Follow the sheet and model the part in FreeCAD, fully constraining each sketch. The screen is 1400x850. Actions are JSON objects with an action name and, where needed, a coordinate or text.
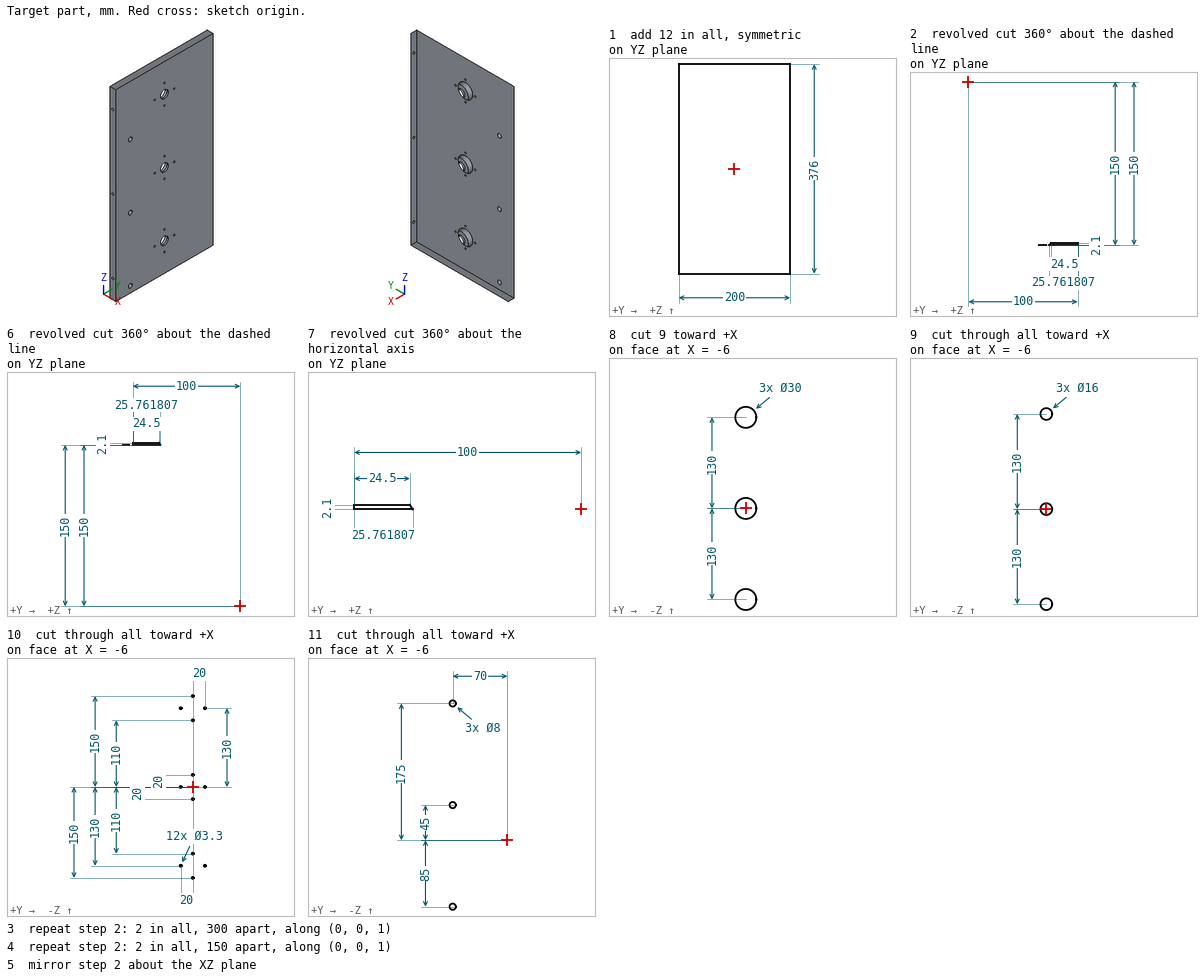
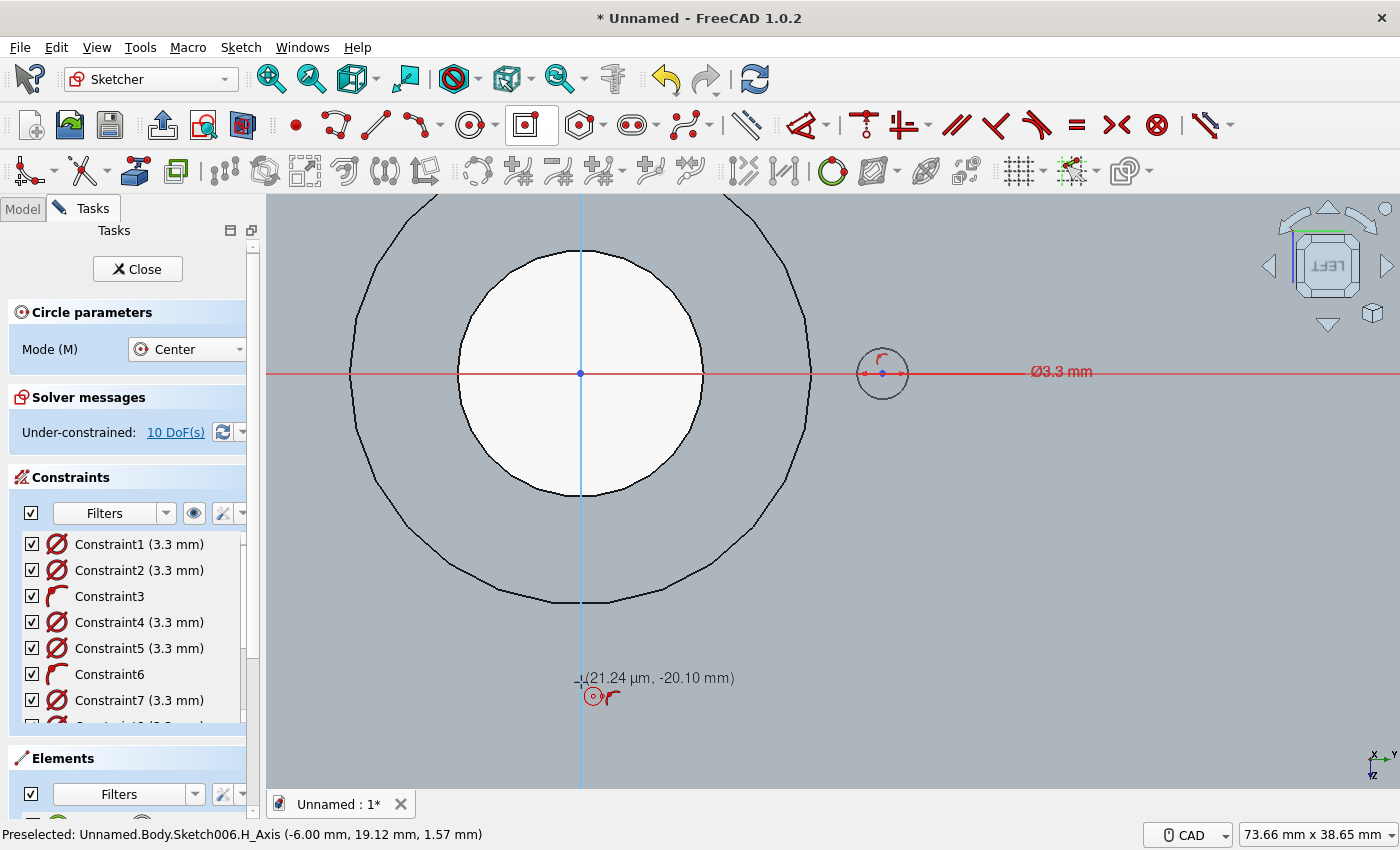
{"action": "scroll", "coordinate": [779, 501], "scroll_direction": "down", "scroll_amount": 13}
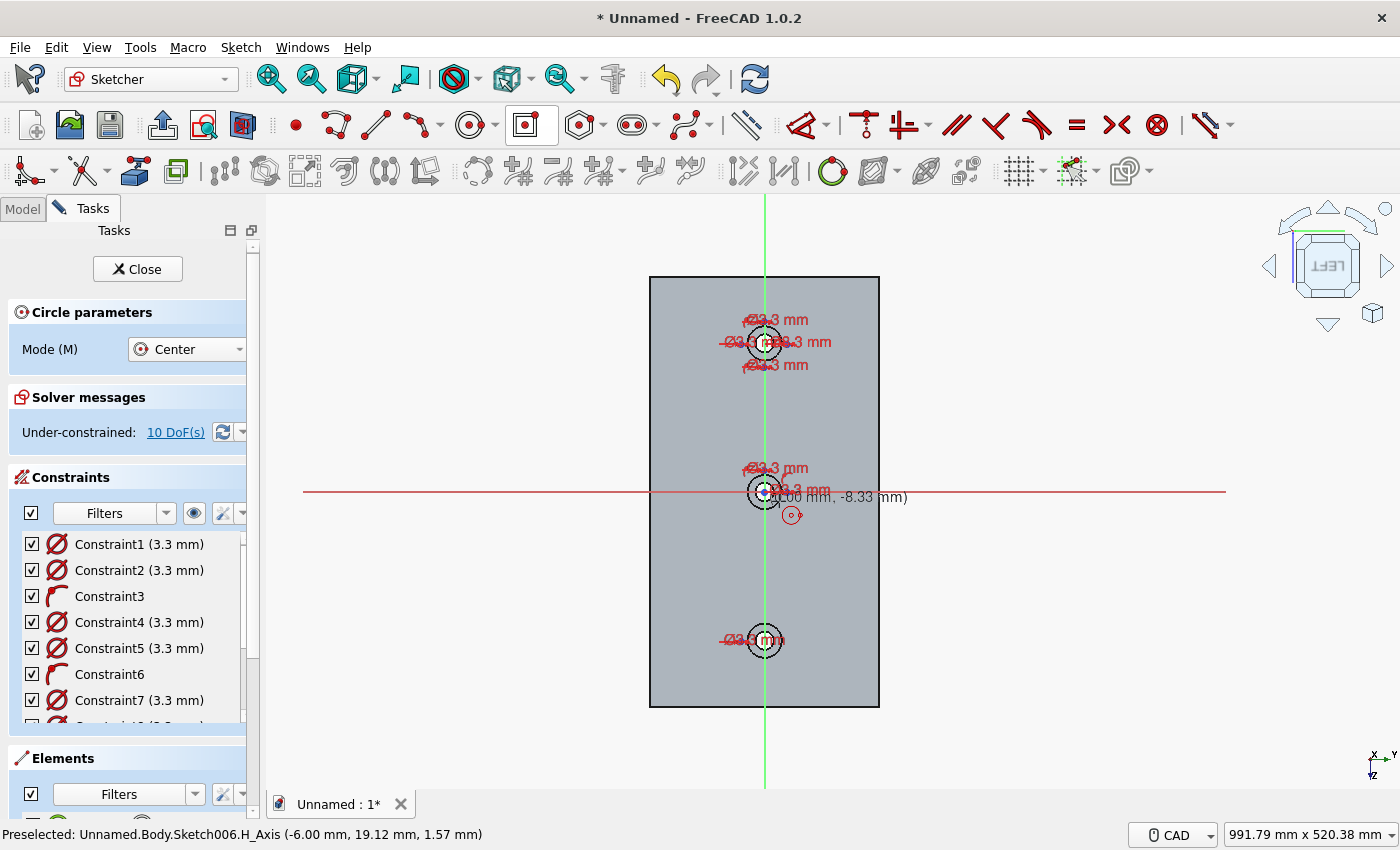
{"action": "left_click", "coordinate": [765, 515]}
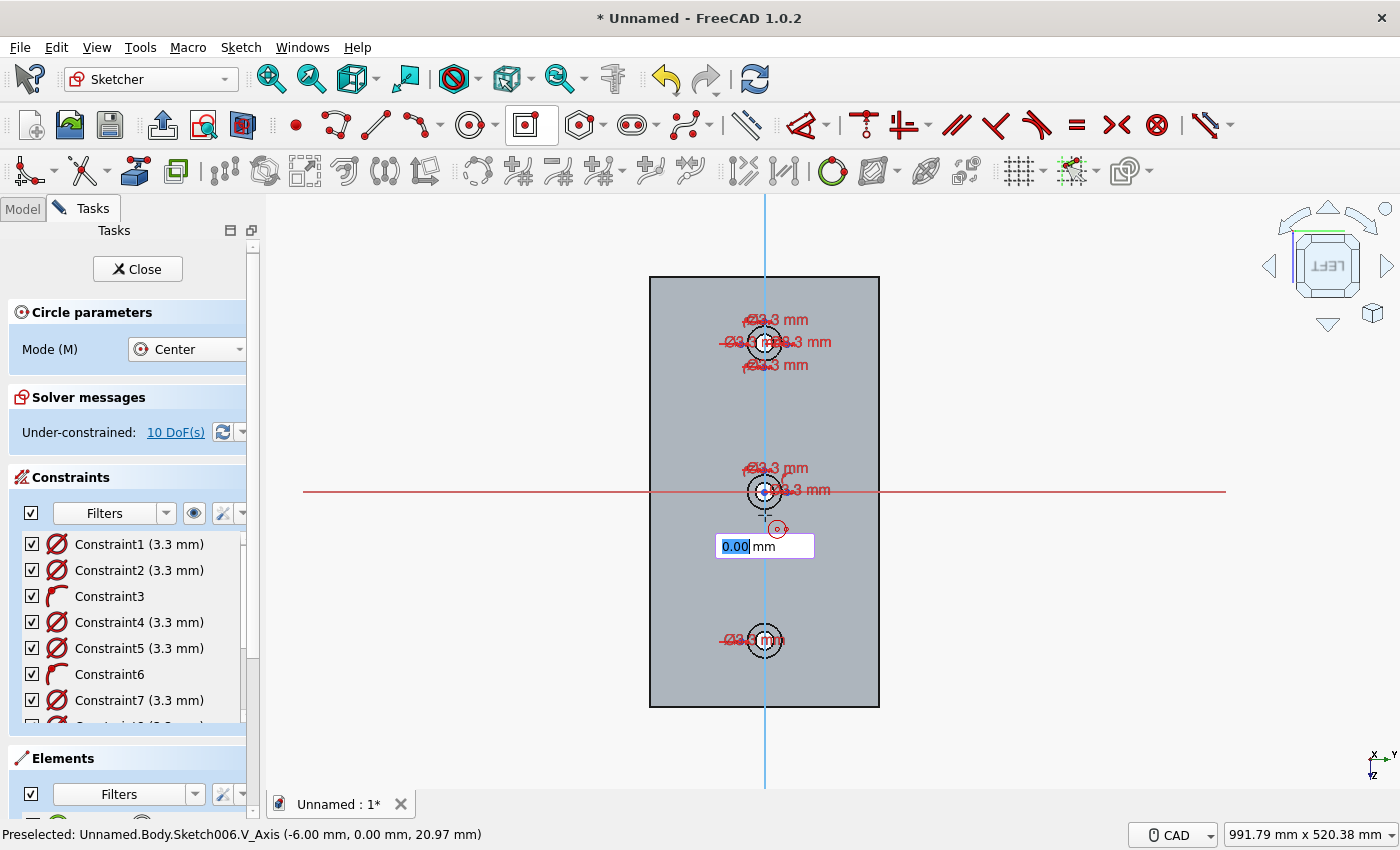
{"action": "scroll", "coordinate": [766, 514], "scroll_direction": "up", "scroll_amount": 11}
{"action": "mouse_move", "coordinate": [767, 512]}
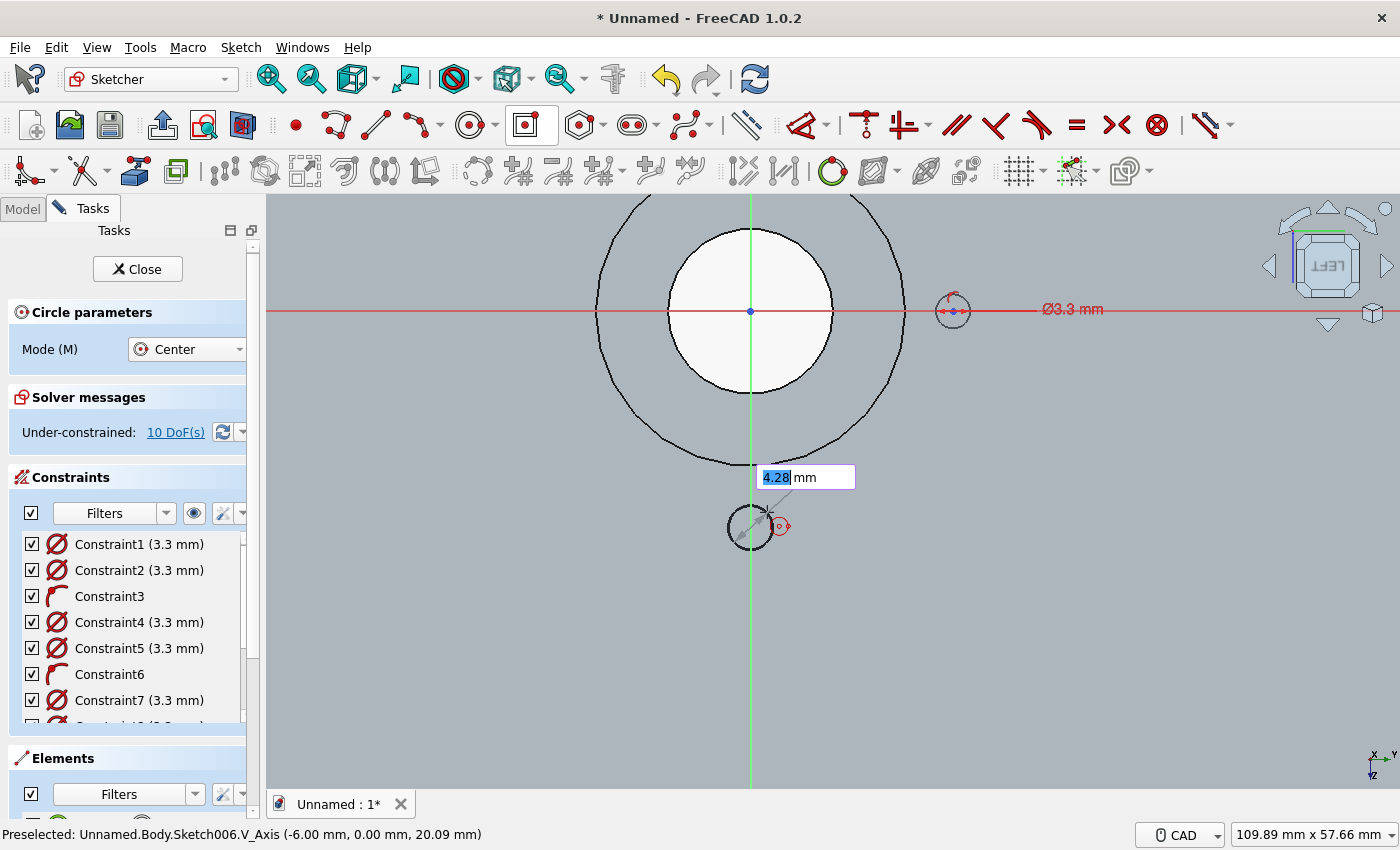
{"action": "type", "text": "3.3"}
{"action": "key", "text": "Return"}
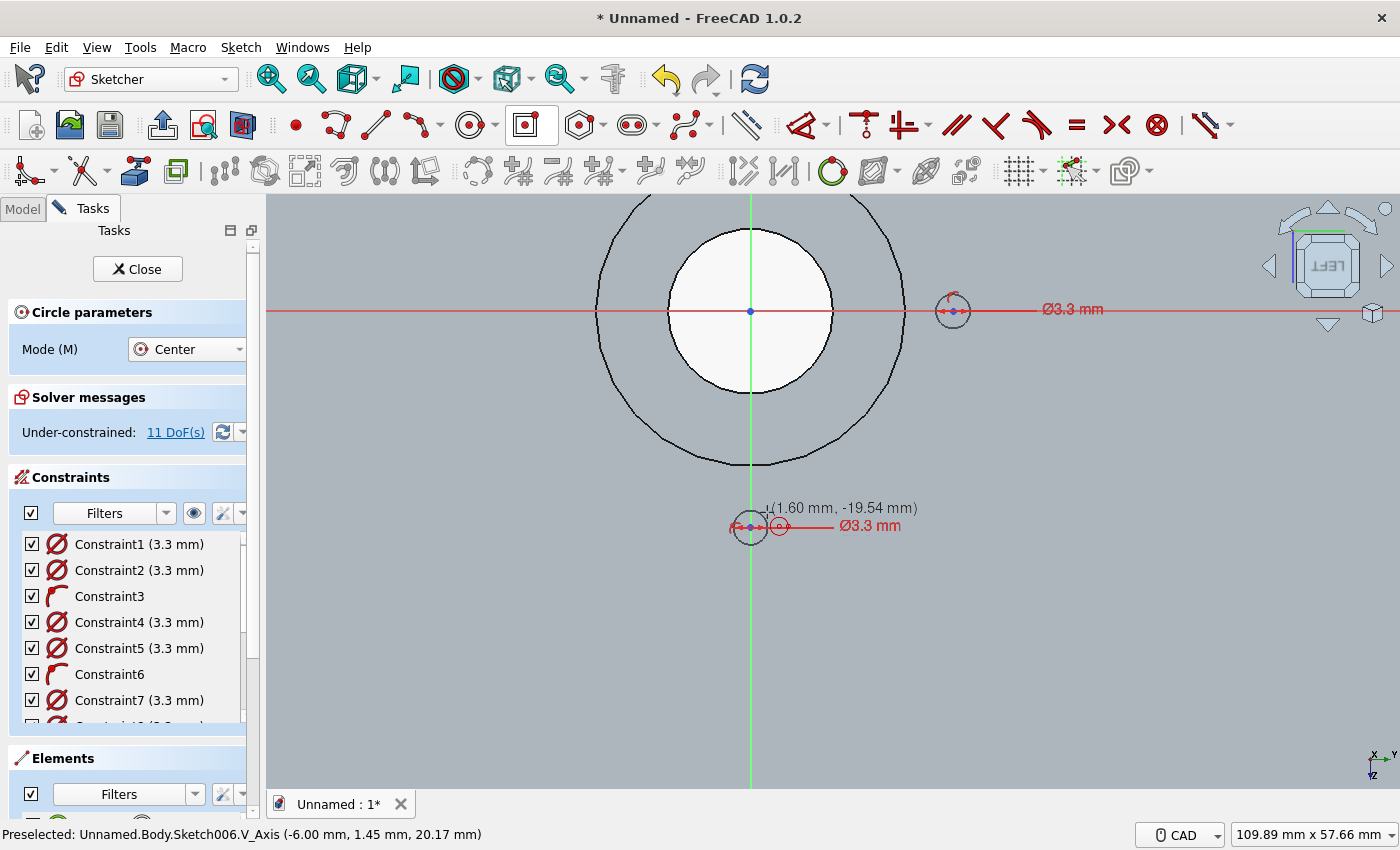
{"action": "scroll", "coordinate": [544, 311], "scroll_direction": "up", "scroll_amount": 2}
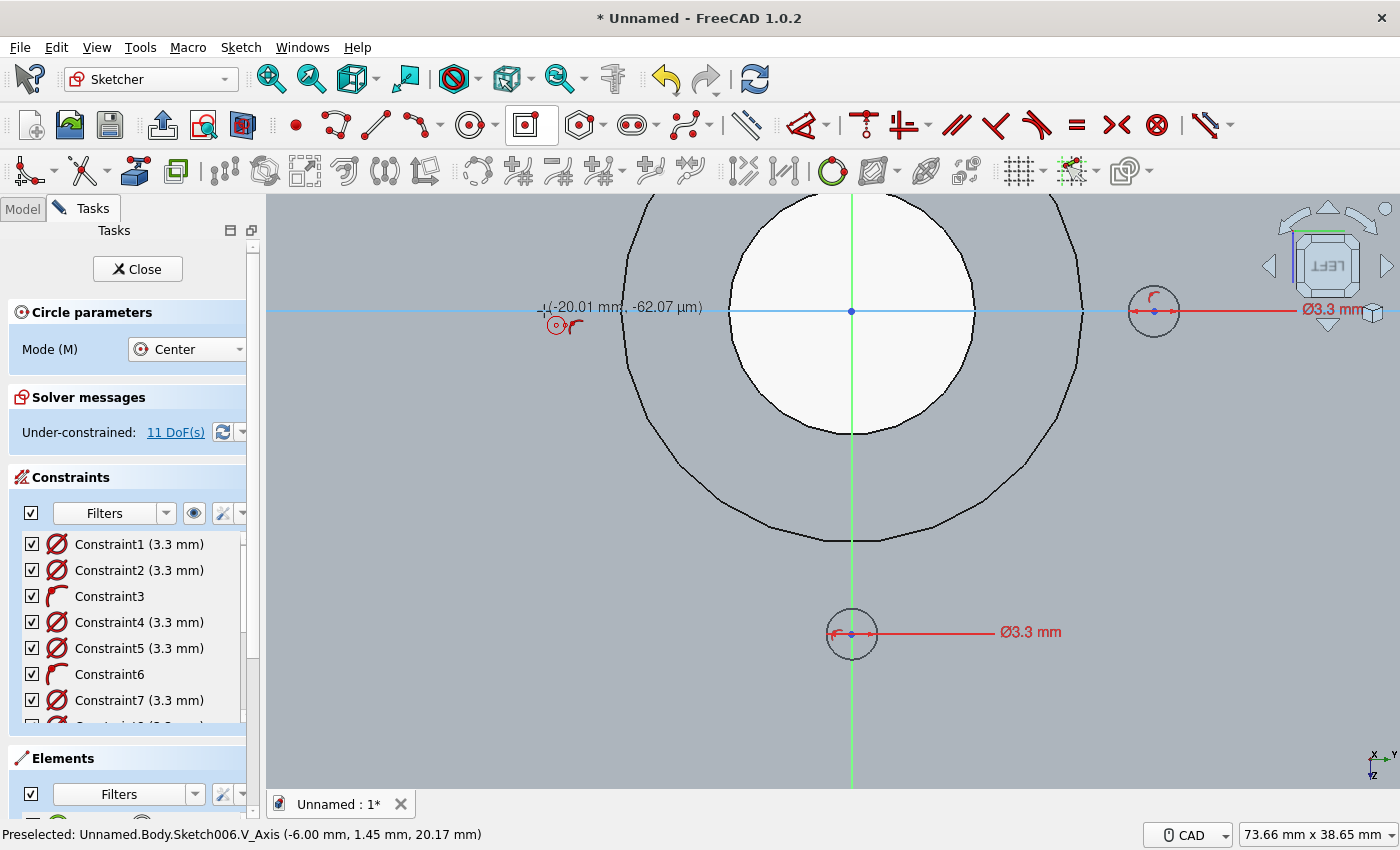
{"action": "scroll", "coordinate": [757, 506], "scroll_direction": "down", "scroll_amount": 13}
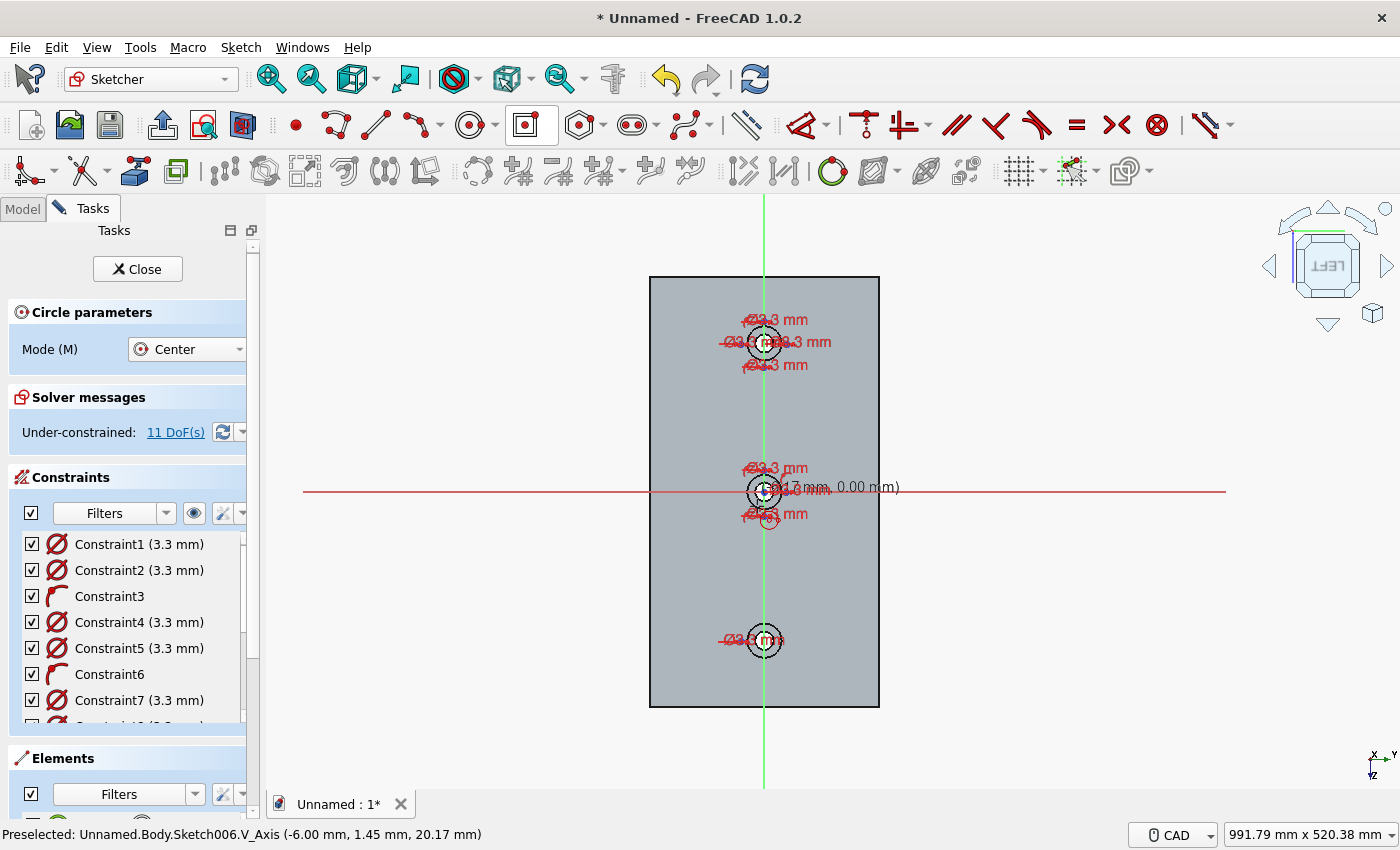
{"action": "left_click", "coordinate": [742, 492]}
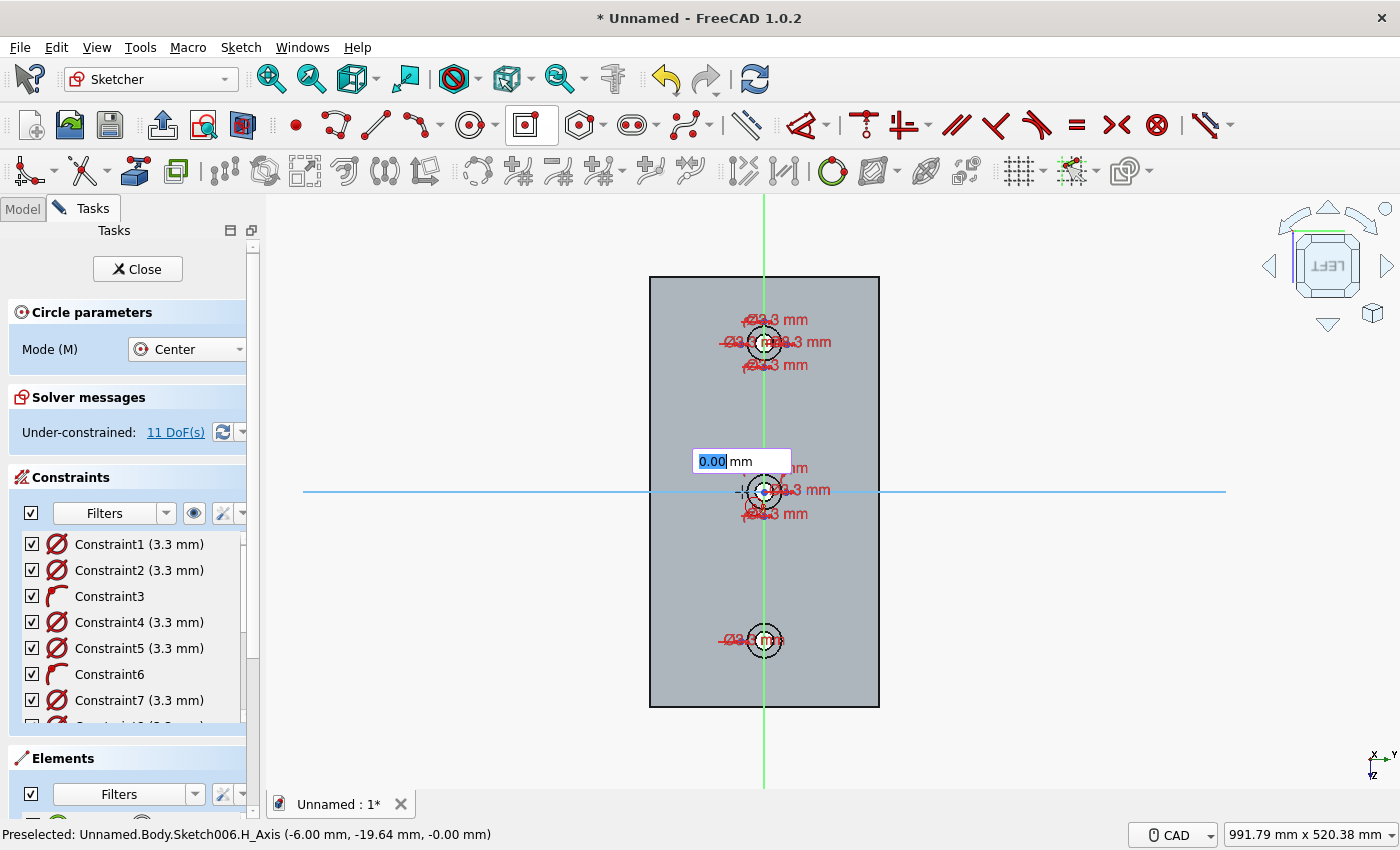
{"action": "scroll", "coordinate": [741, 494], "scroll_direction": "up", "scroll_amount": 11}
{"action": "mouse_move", "coordinate": [737, 488]}